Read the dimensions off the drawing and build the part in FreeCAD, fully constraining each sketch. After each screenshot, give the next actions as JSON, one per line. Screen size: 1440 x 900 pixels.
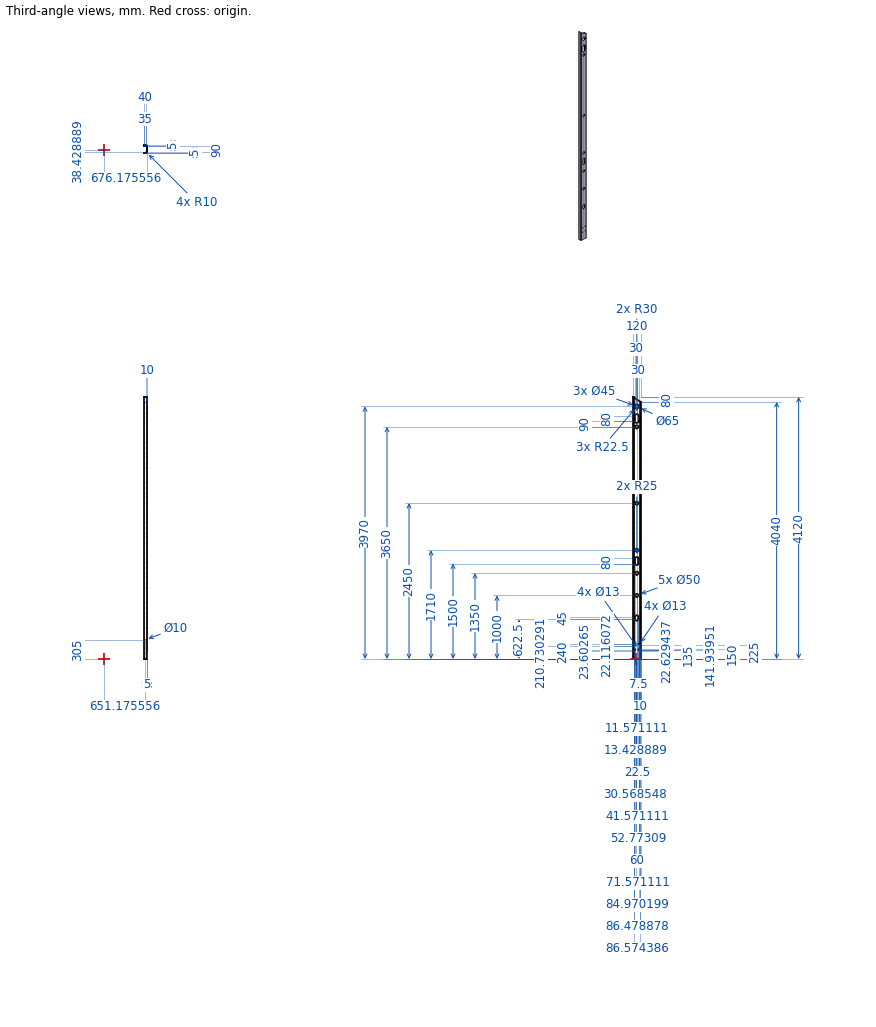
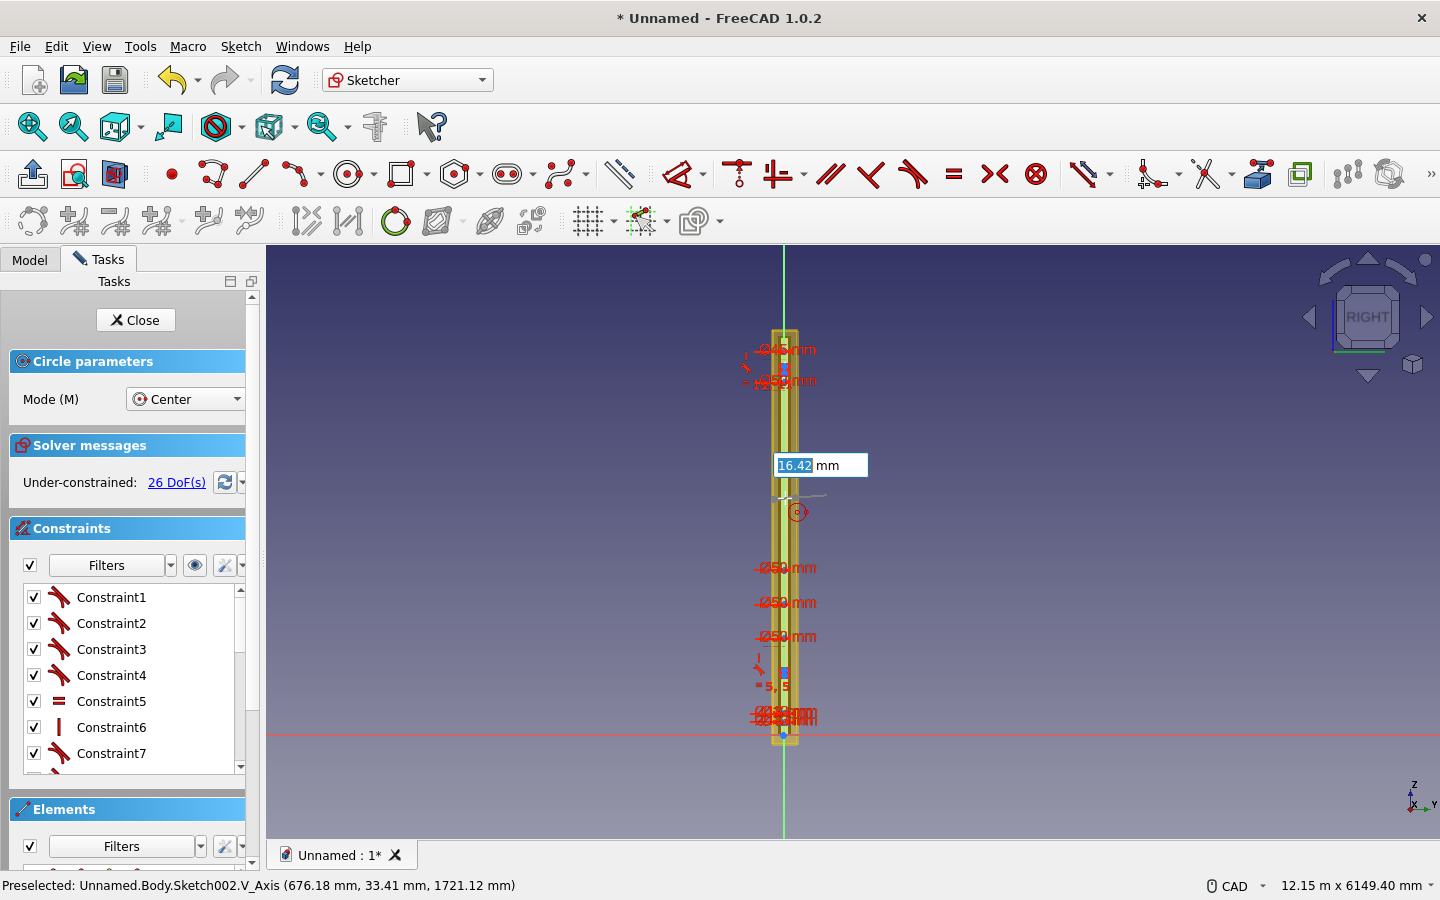
{"action": "scroll", "coordinate": [786, 497], "scroll_direction": "up", "scroll_amount": 9}
{"action": "mouse_move", "coordinate": [786, 493]}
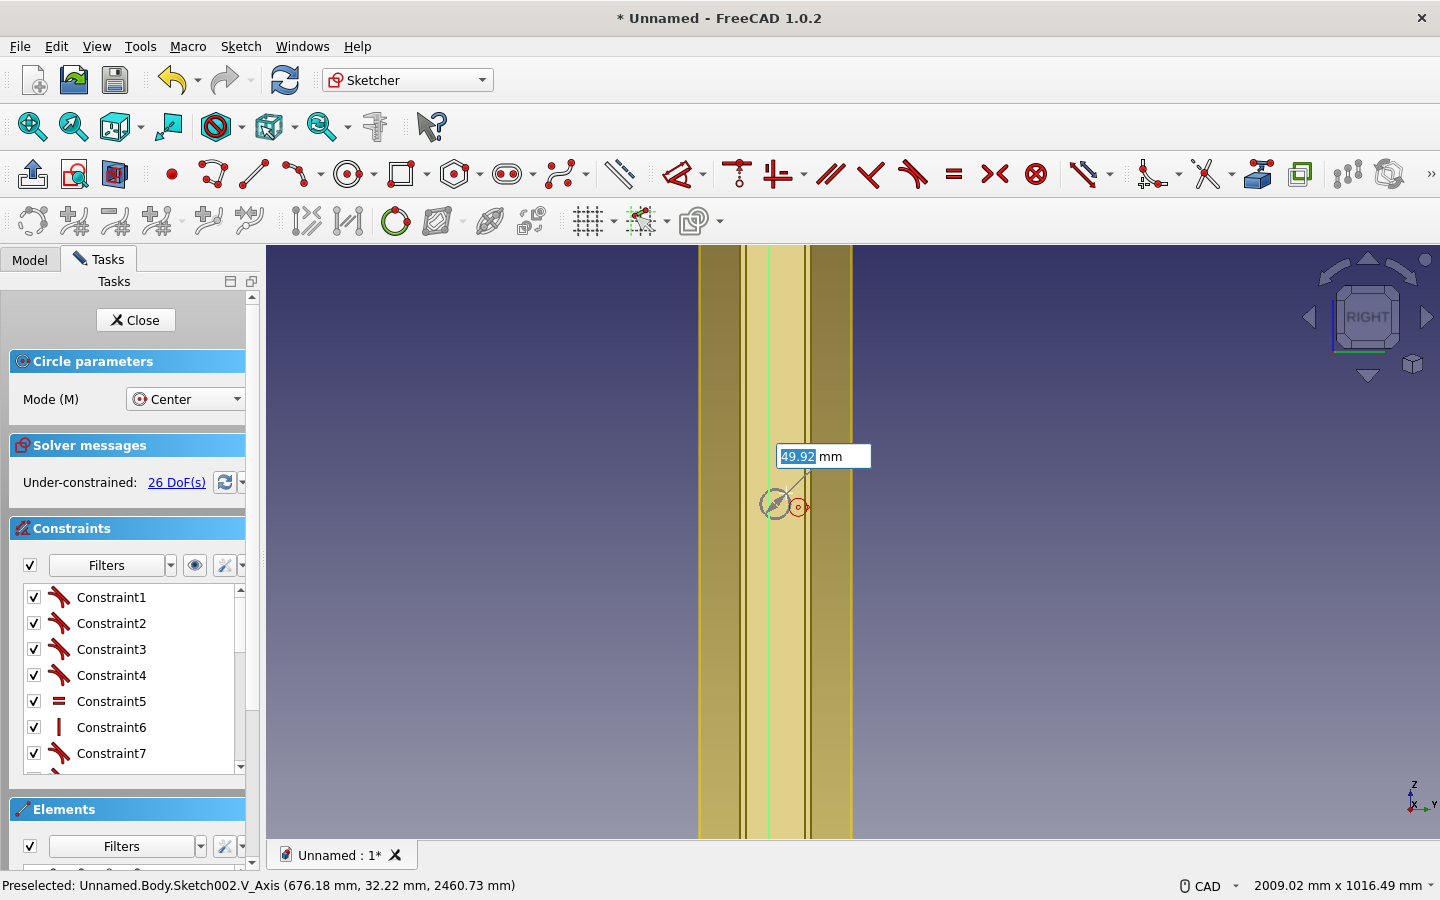
{"action": "type", "text": "50"}
{"action": "key", "text": "Return"}
{"action": "key", "text": "Escape"}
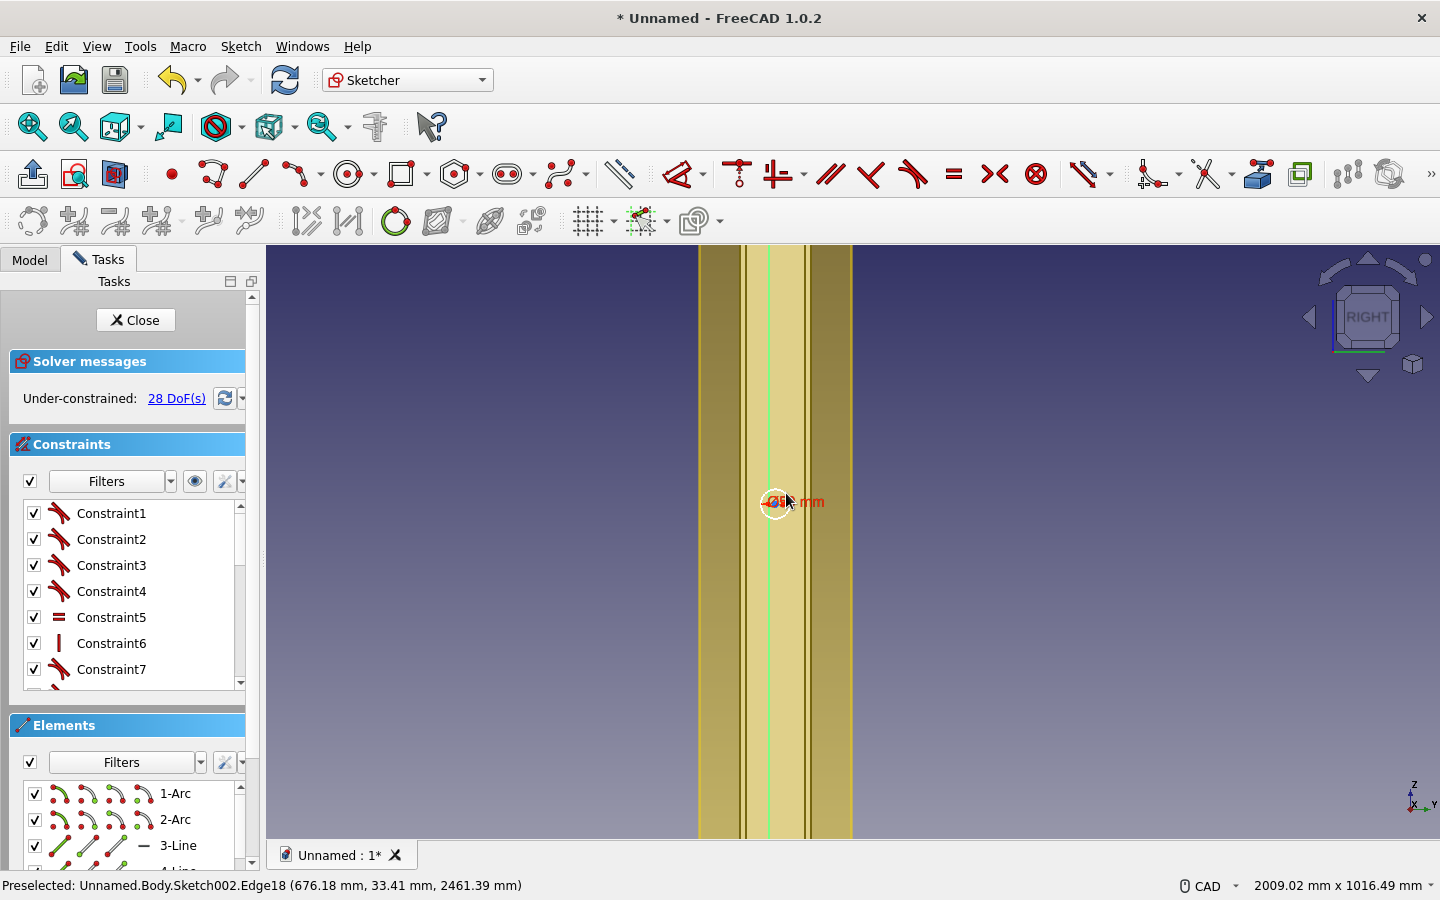
{"action": "scroll", "coordinate": [786, 497], "scroll_direction": "down", "scroll_amount": 9}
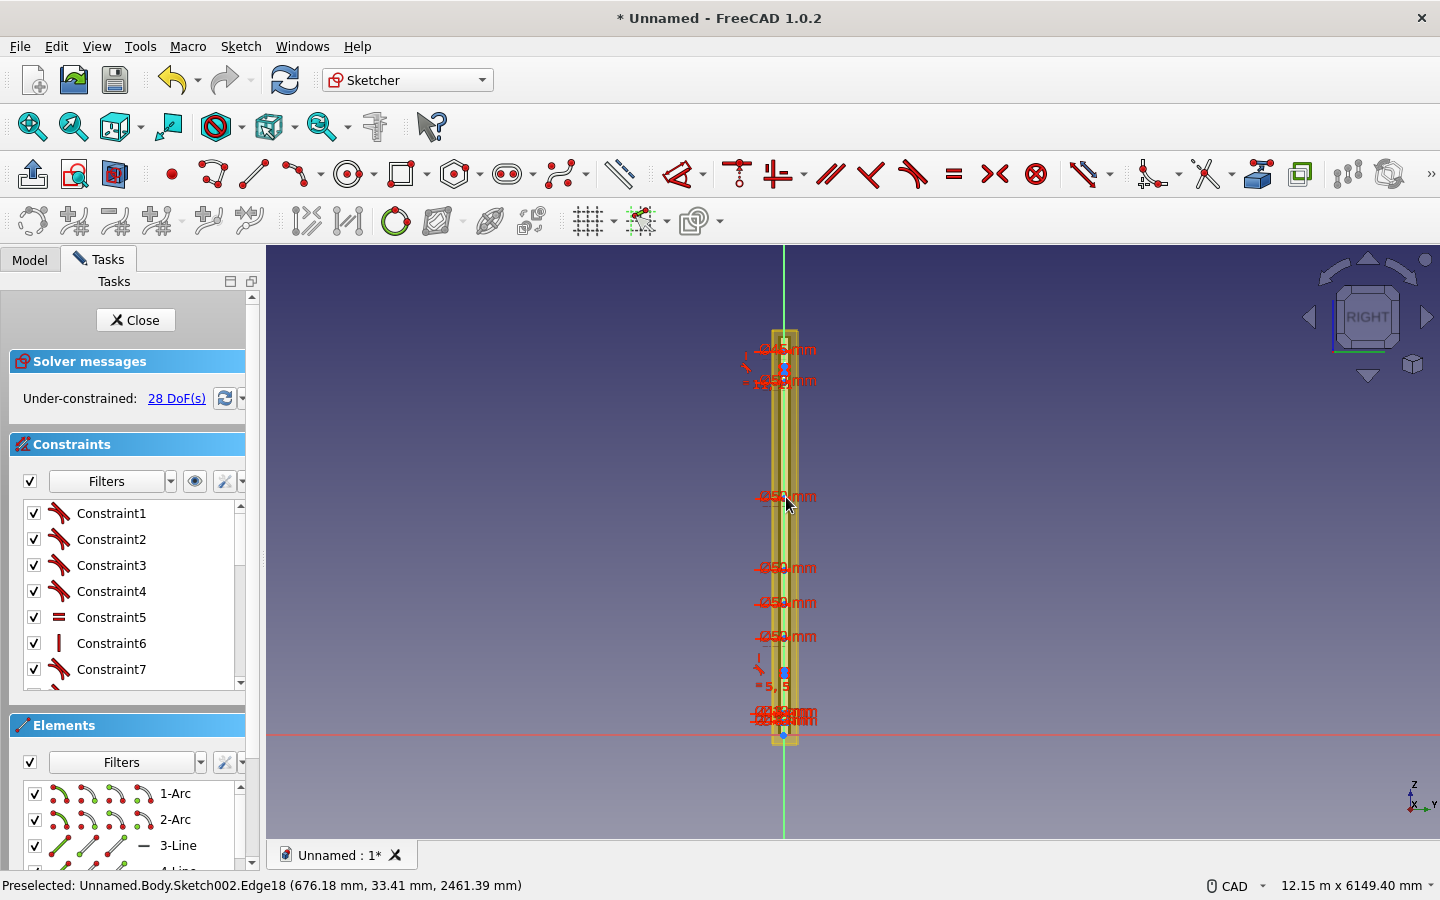
{"action": "scroll", "coordinate": [787, 714], "scroll_direction": "up", "scroll_amount": 4}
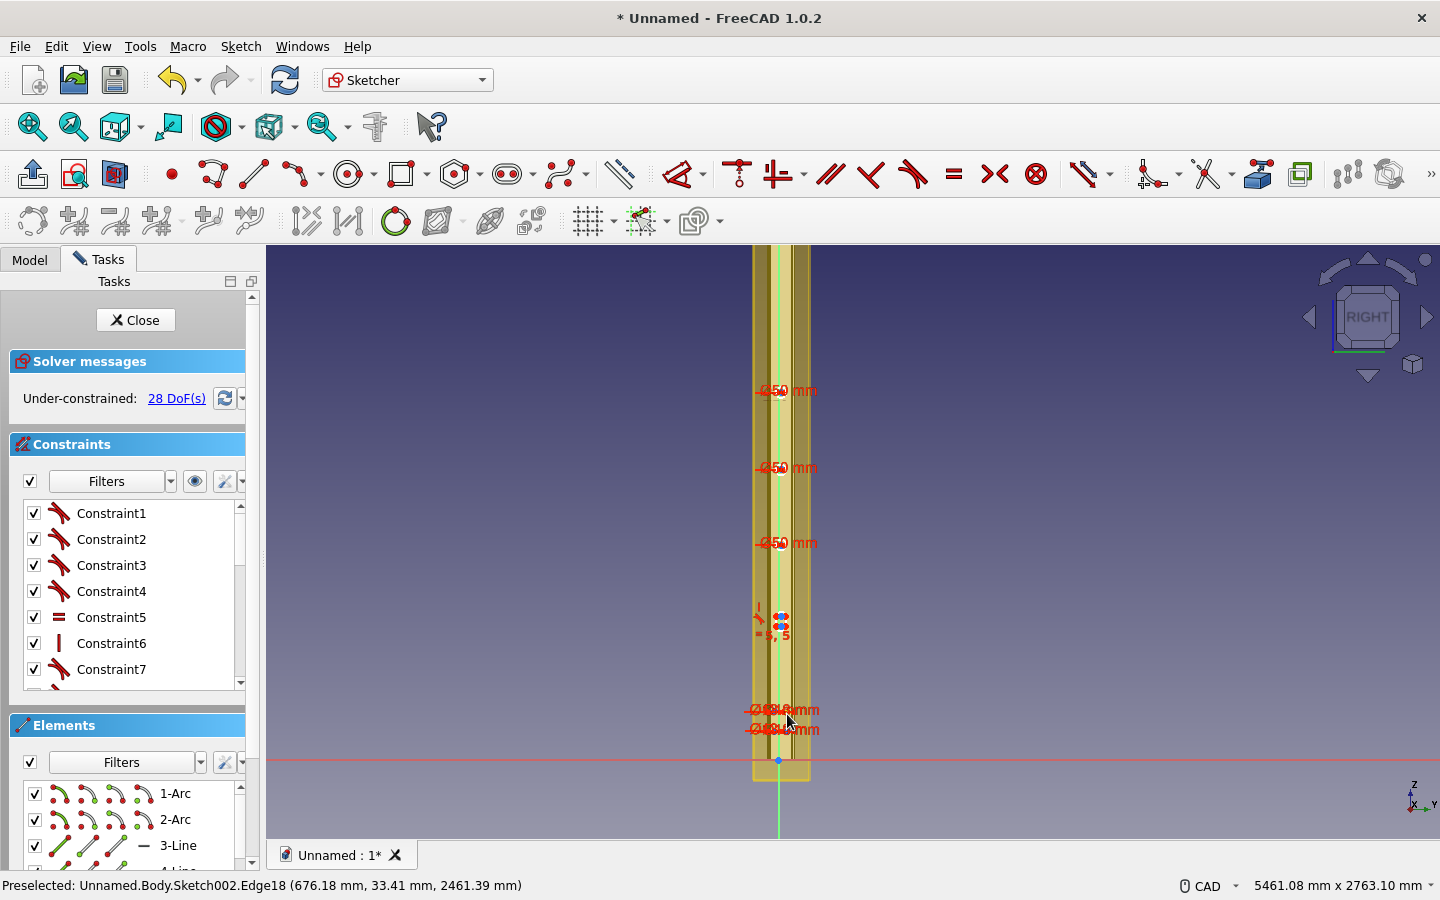
{"action": "left_click", "coordinate": [787, 712]}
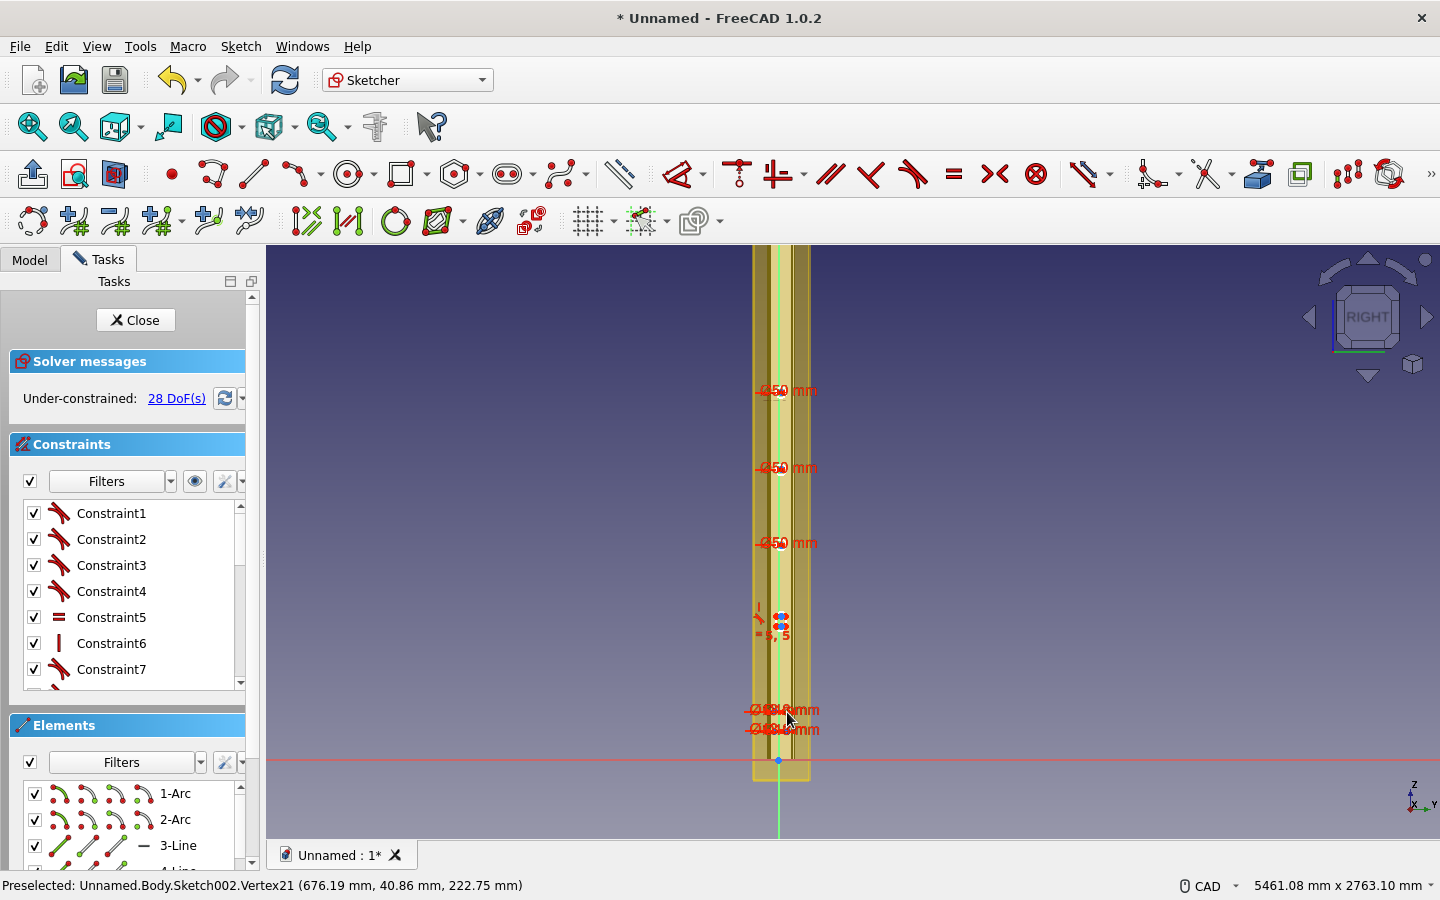
{"action": "left_click", "coordinate": [787, 732]}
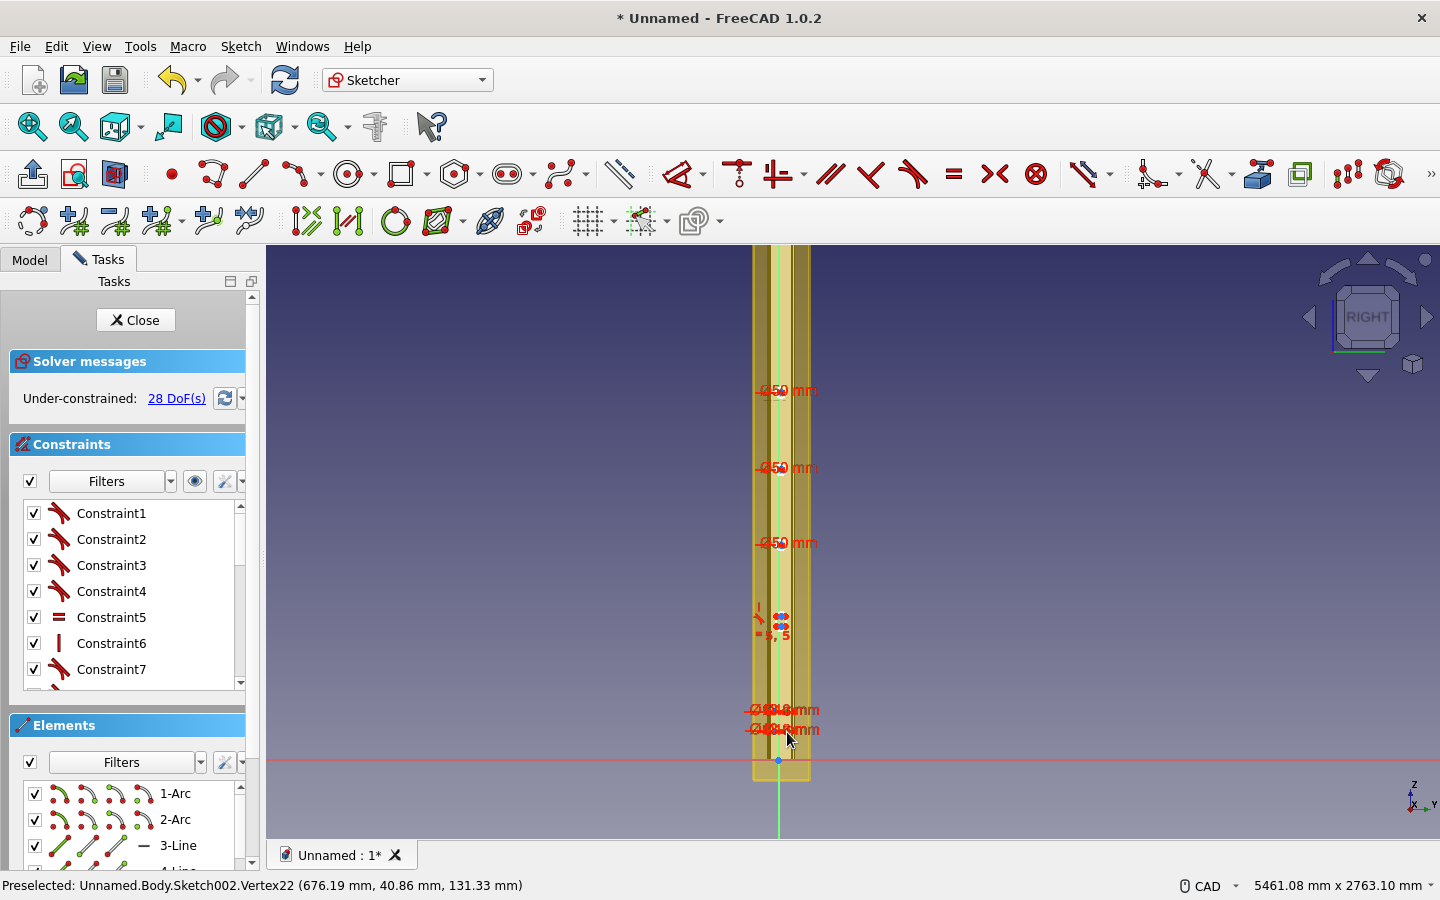
{"action": "left_click", "coordinate": [804, 174]}